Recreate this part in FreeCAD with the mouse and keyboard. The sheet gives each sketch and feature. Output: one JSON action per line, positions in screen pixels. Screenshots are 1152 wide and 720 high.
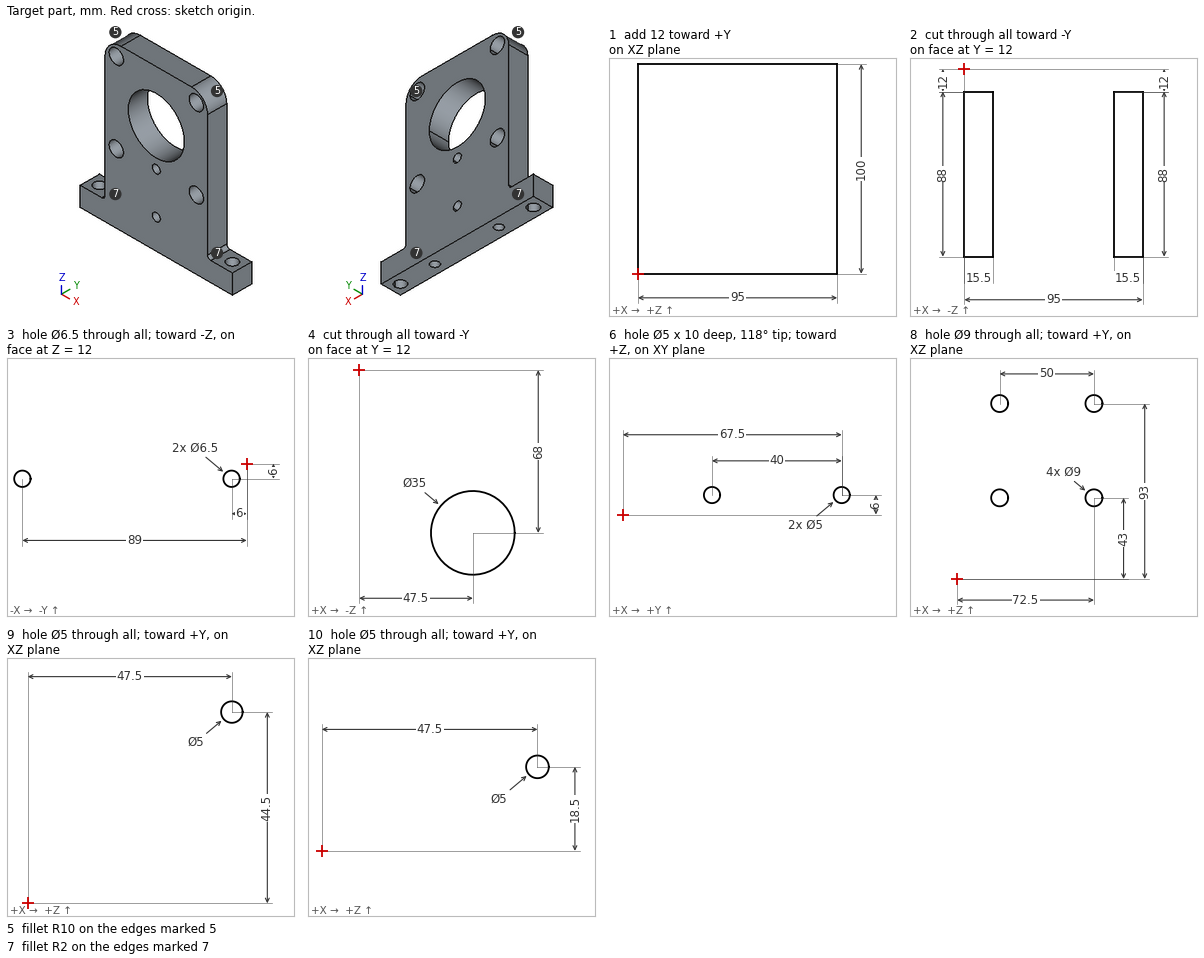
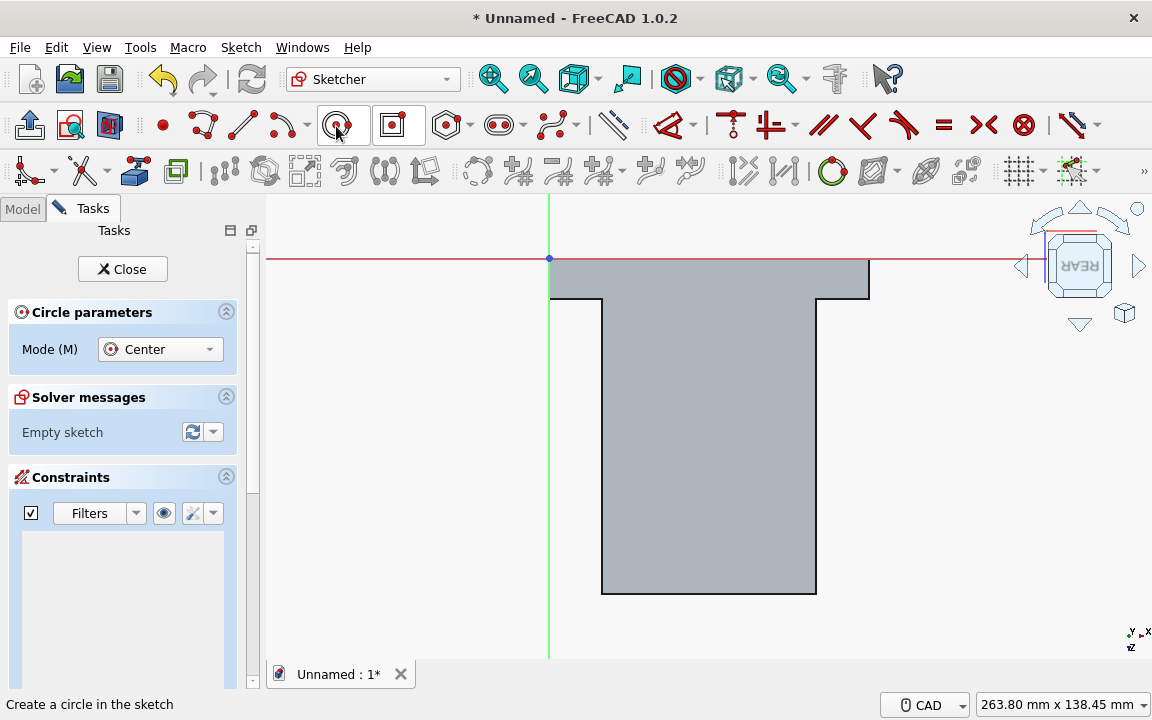
{"action": "left_click", "coordinate": [709, 487]}
{"action": "left_click", "coordinate": [751, 445]}
{"action": "key", "text": "Escape"}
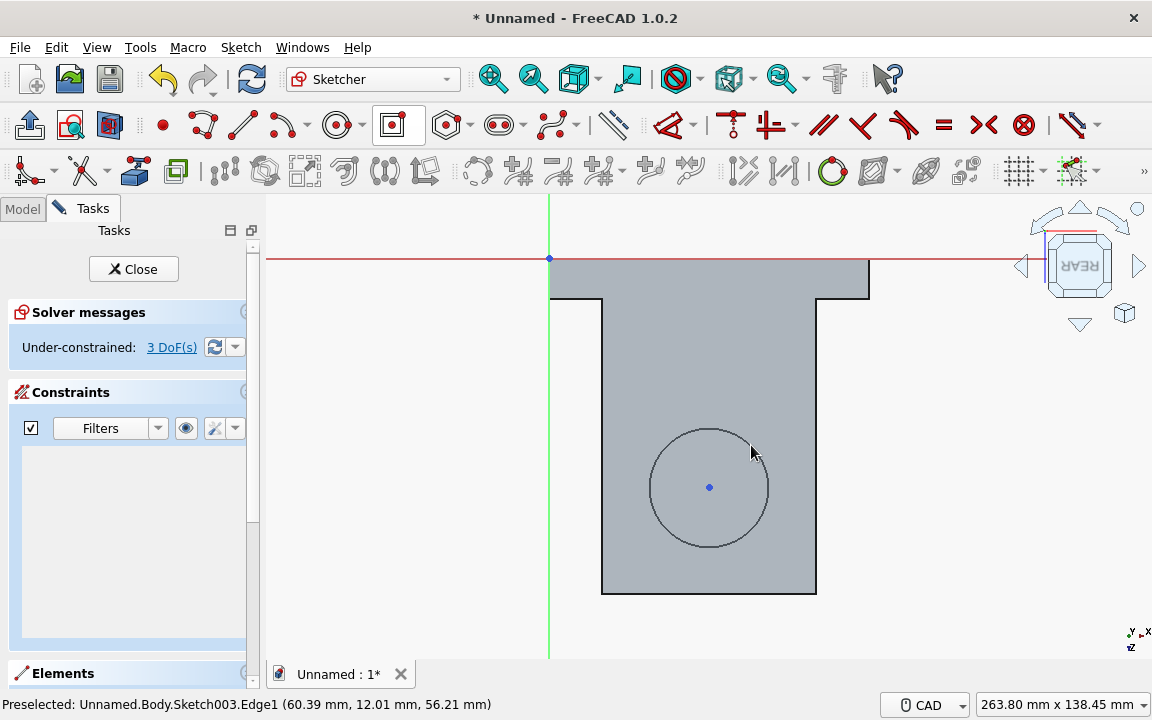
{"action": "left_click", "coordinate": [668, 126]}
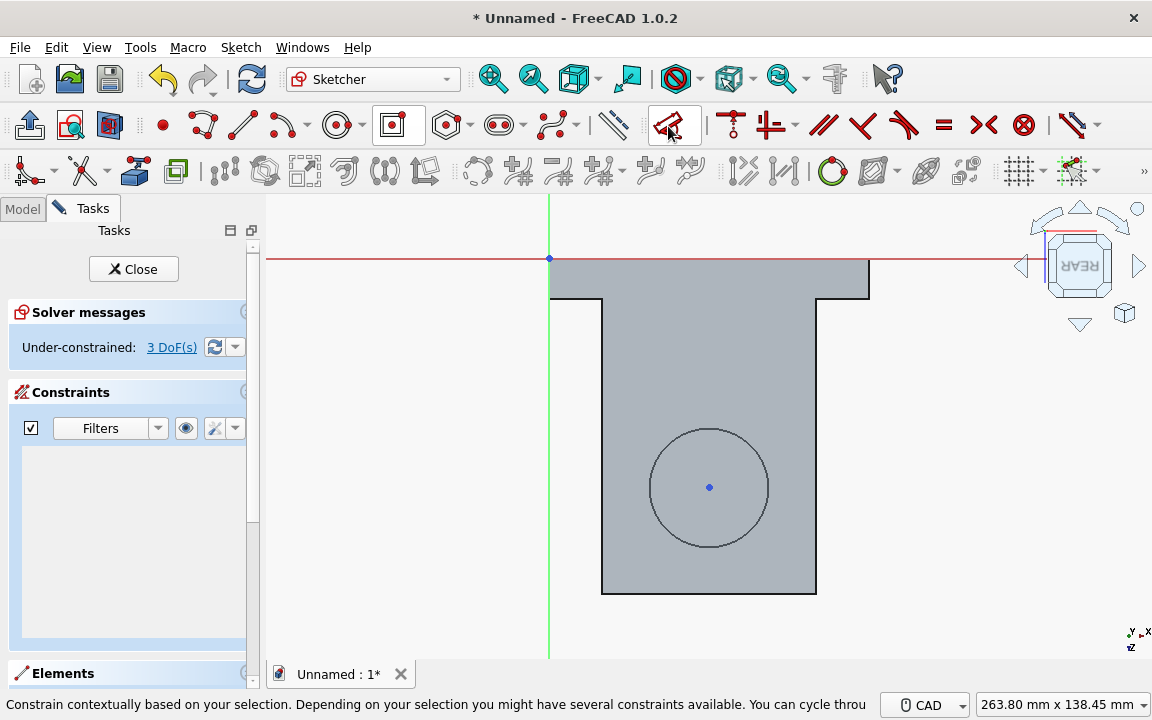
{"action": "left_click", "coordinate": [751, 446]}
{"action": "left_click", "coordinate": [774, 423]}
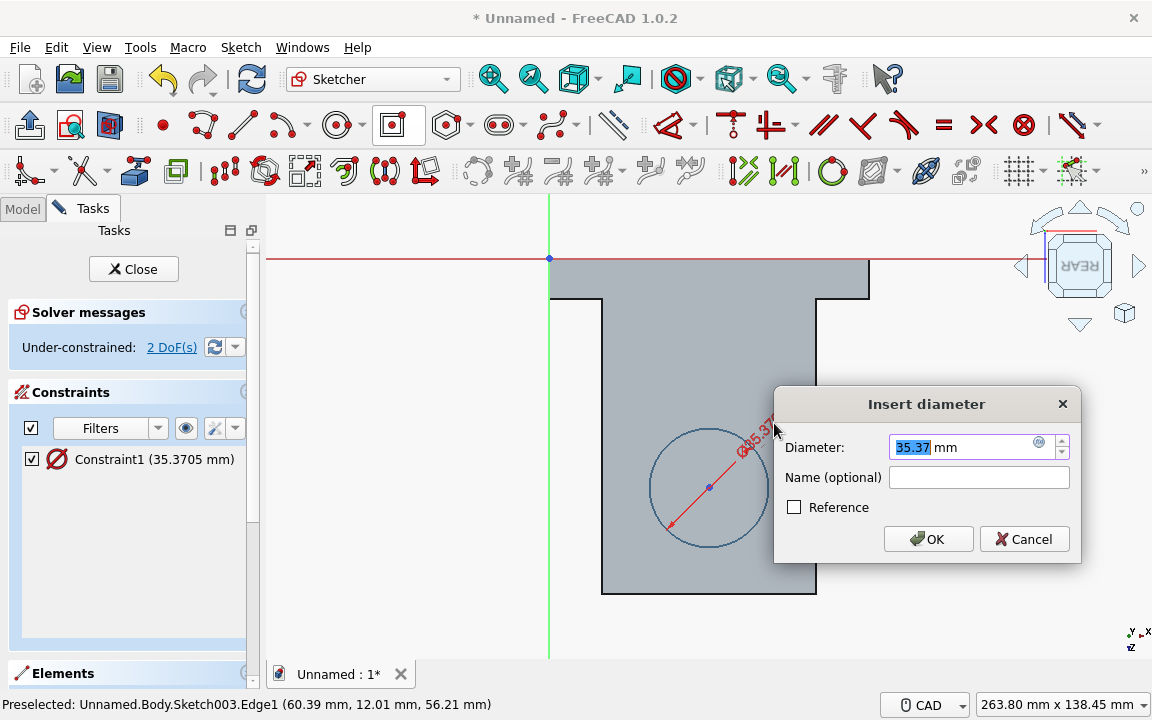
{"action": "type", "text": "35"}
{"action": "key", "text": "Return"}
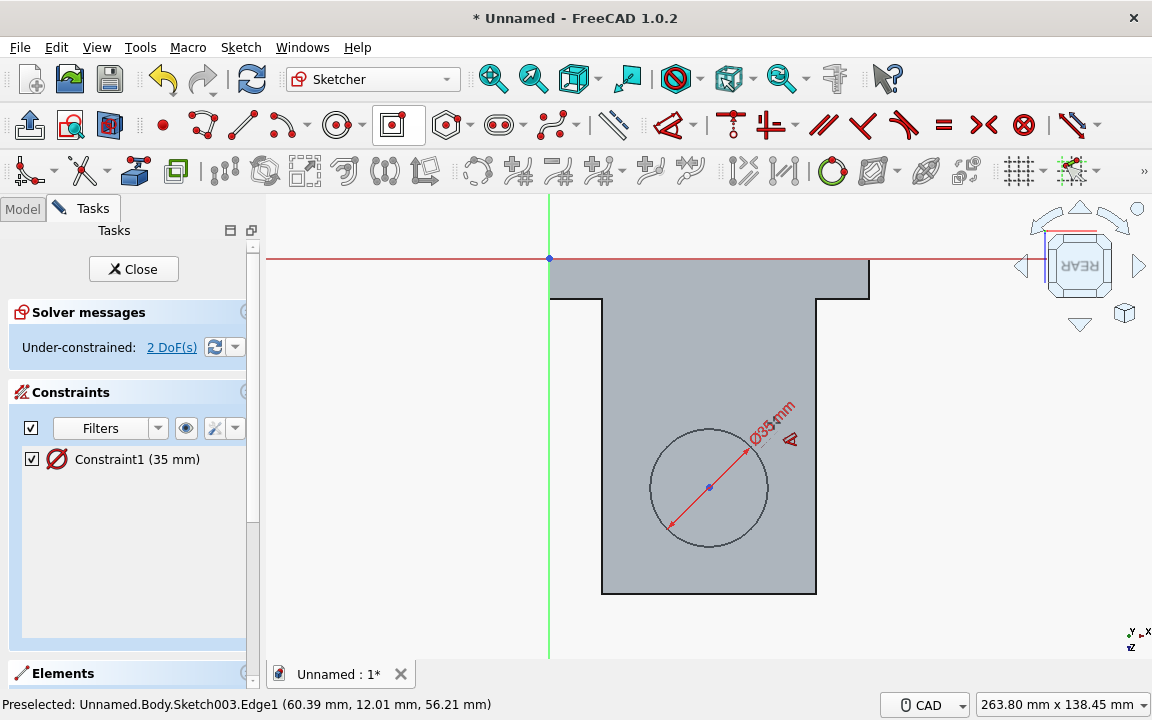
{"action": "left_click", "coordinate": [709, 488]}
{"action": "left_click", "coordinate": [515, 373]}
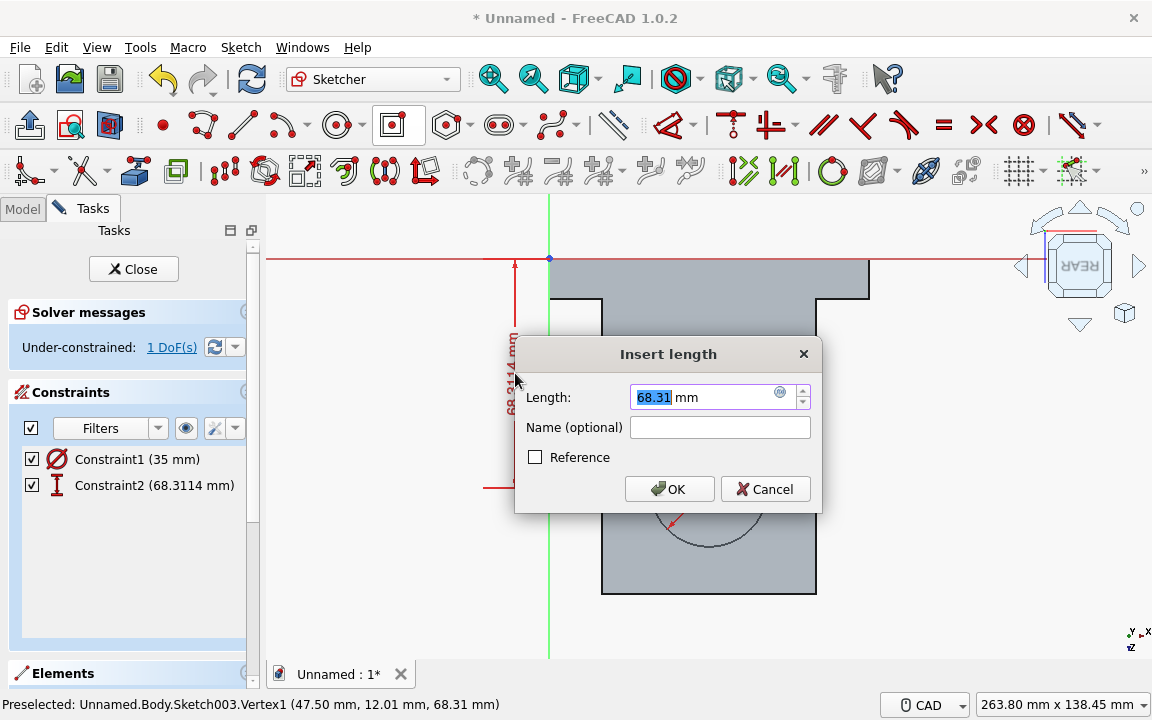
{"action": "type", "text": "68"}
{"action": "key", "text": "Return"}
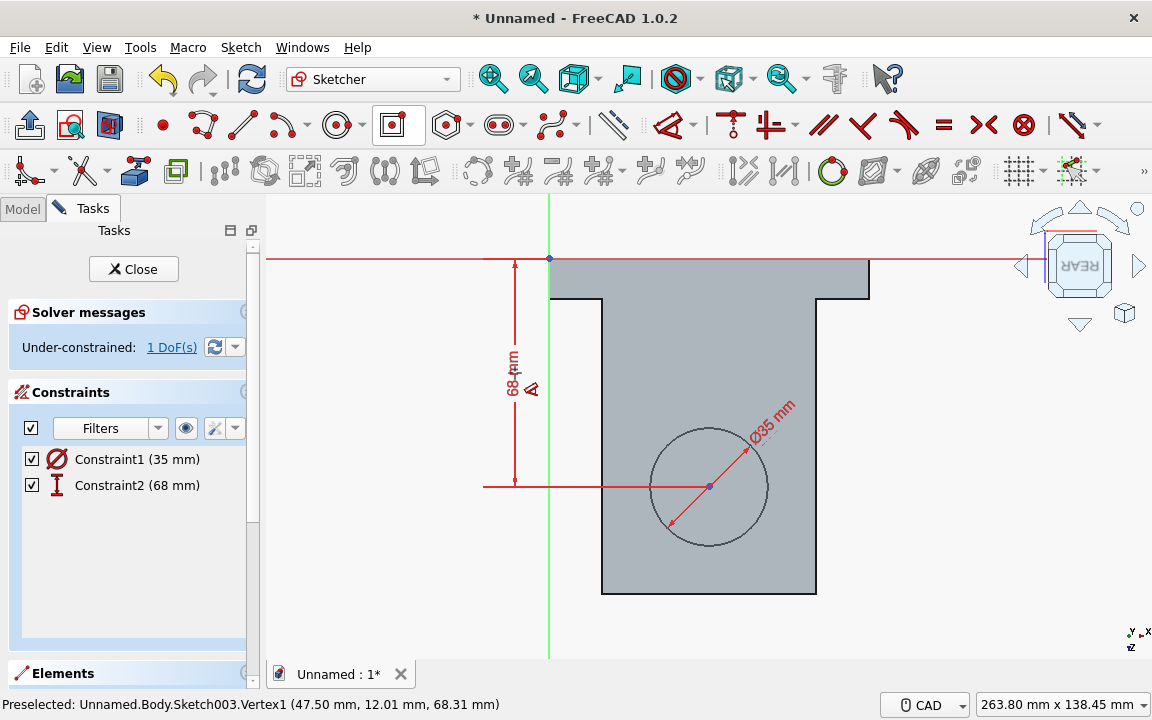
{"action": "left_click", "coordinate": [709, 487]}
{"action": "left_click", "coordinate": [629, 225]}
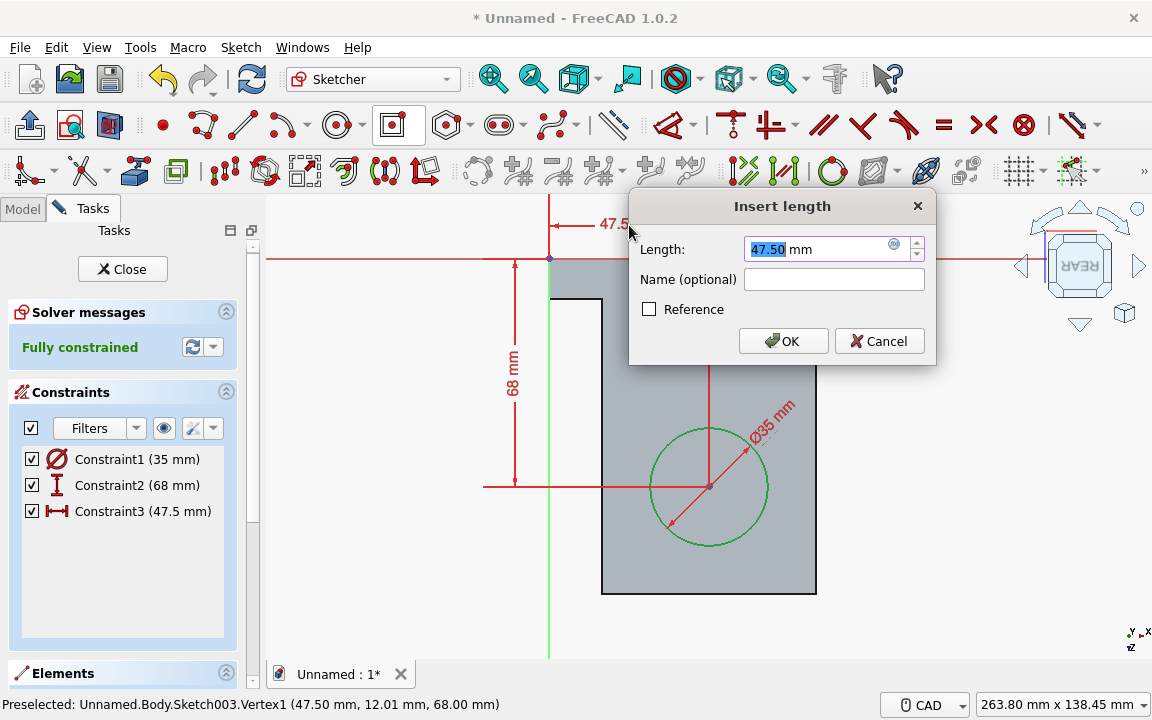
{"action": "type", "text": "47.5"}
{"action": "key", "text": "Return"}
{"action": "key", "text": "Escape"}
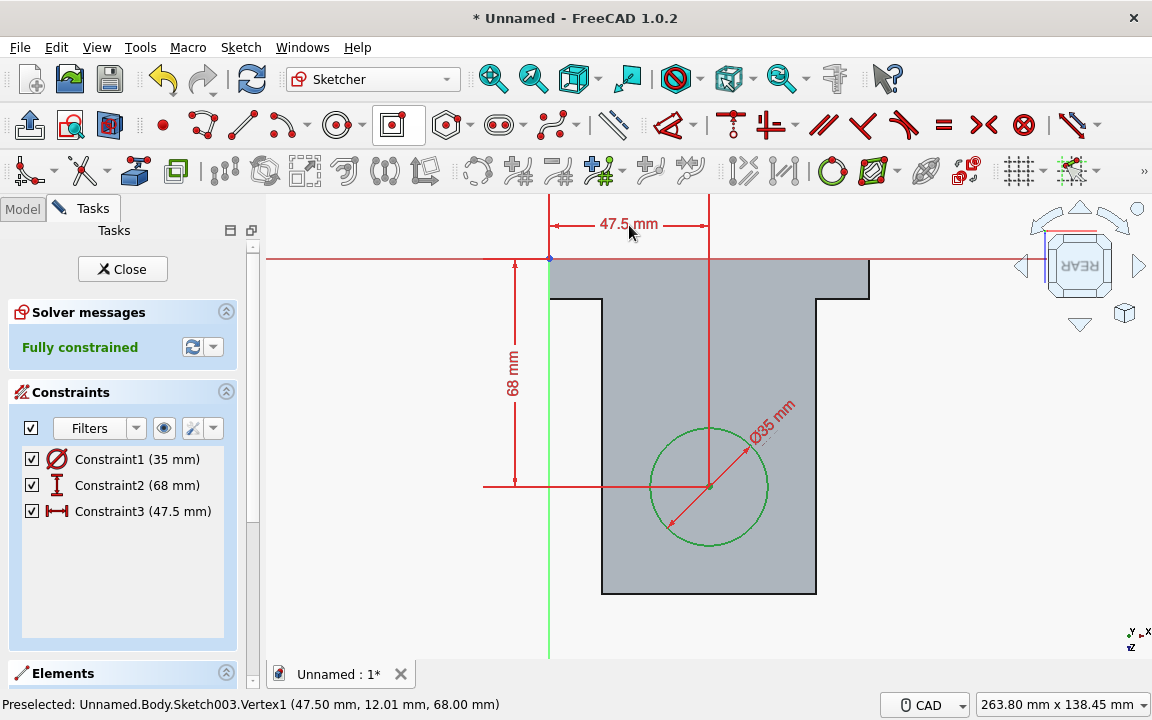
{"action": "left_click", "coordinate": [123, 269]}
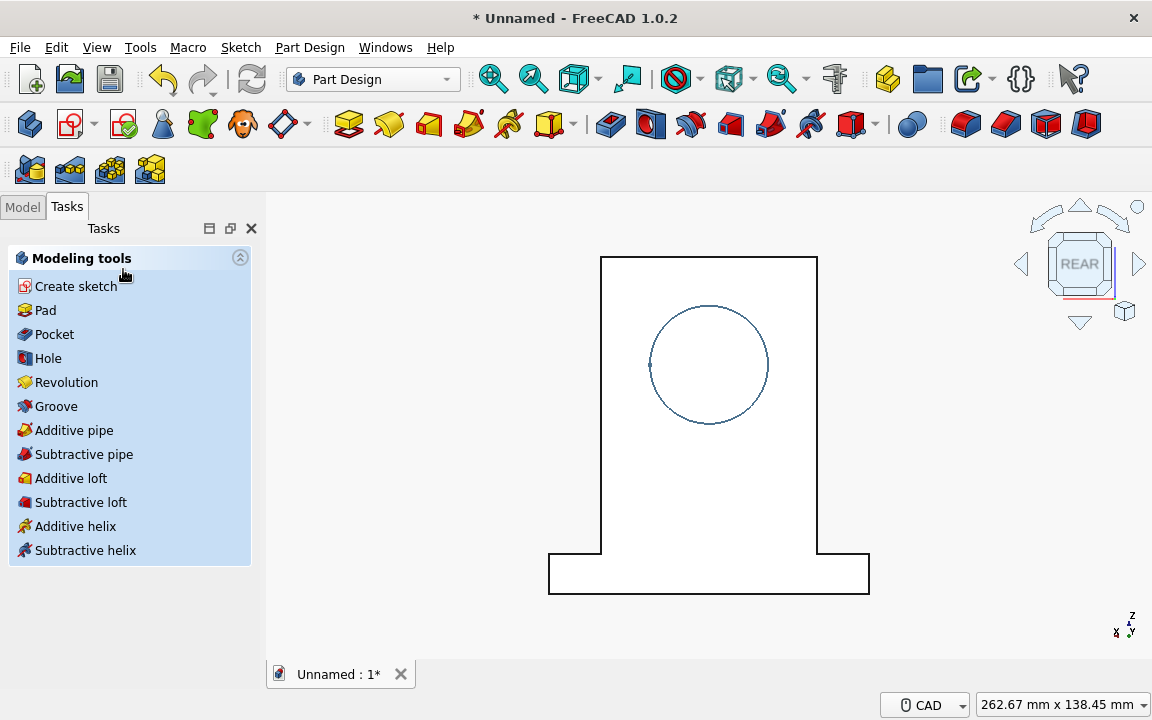
{"action": "left_click", "coordinate": [612, 124]}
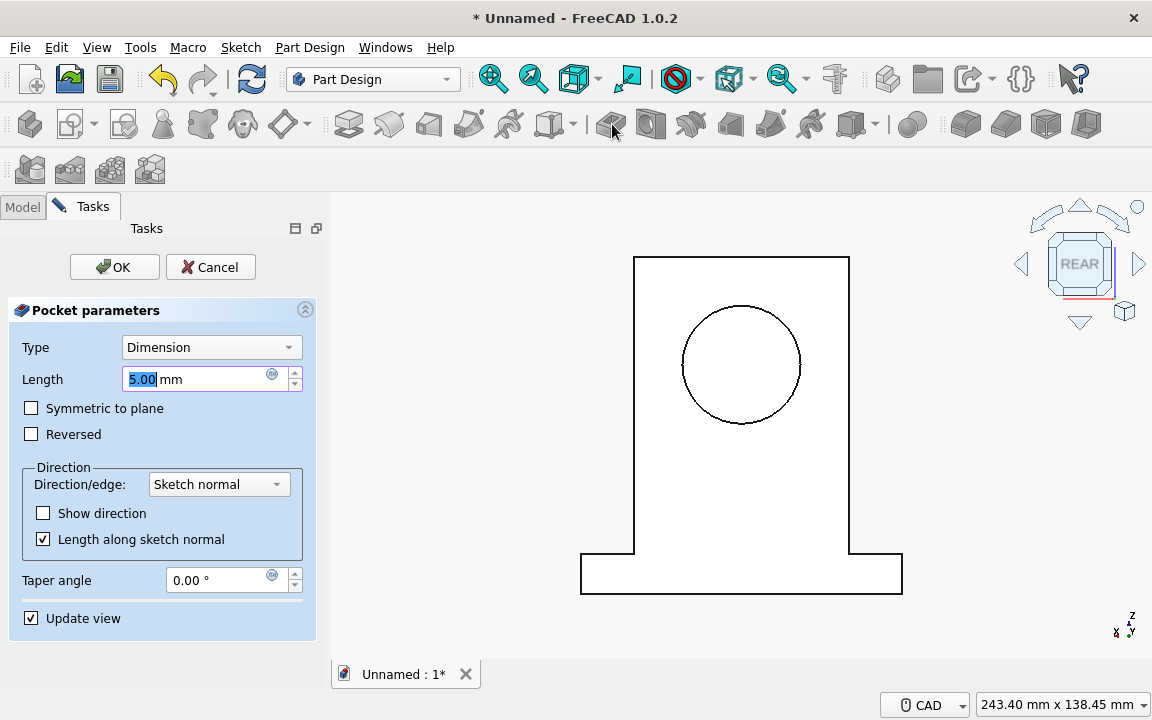
{"action": "left_click", "coordinate": [212, 348]}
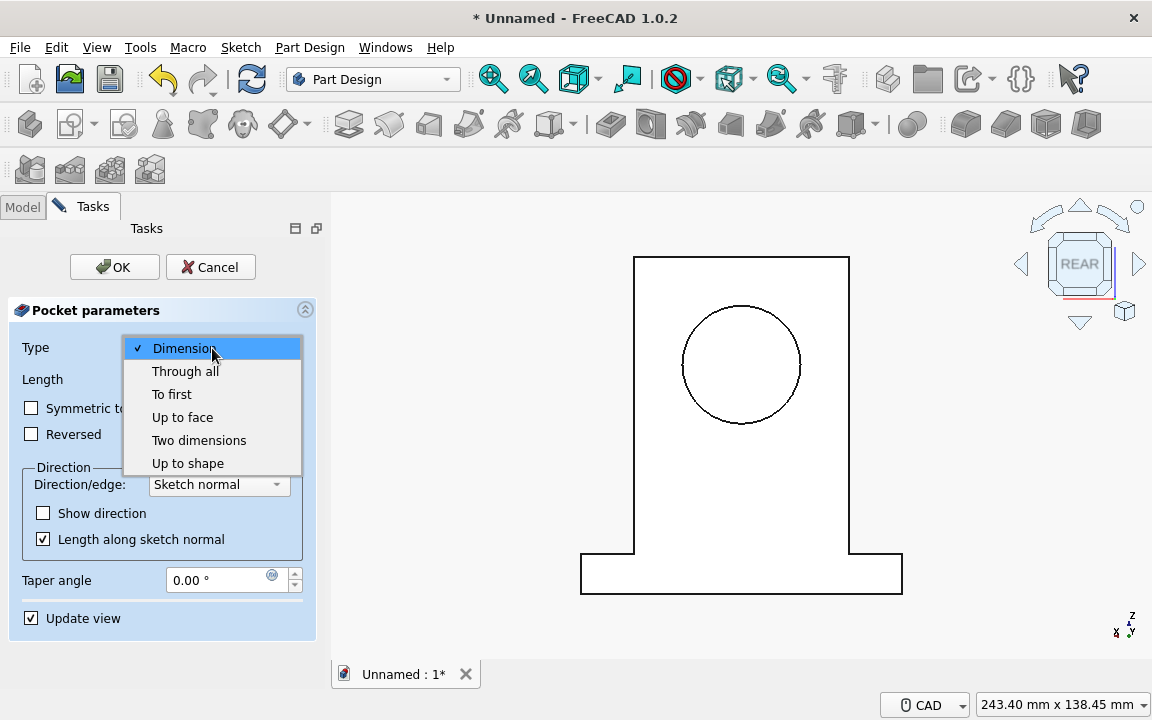
{"action": "left_click", "coordinate": [212, 372]}